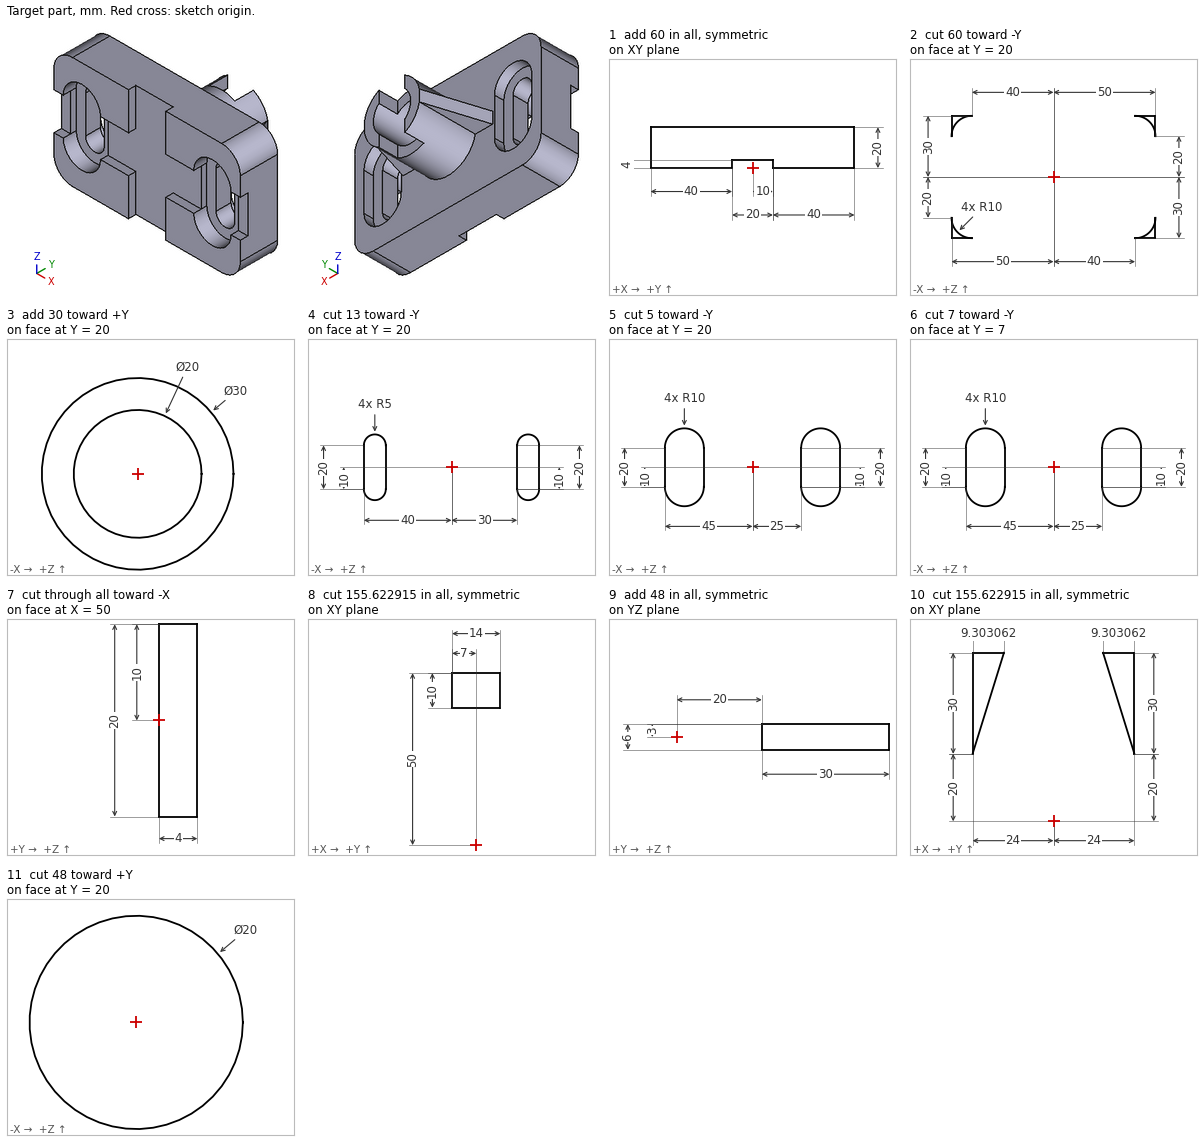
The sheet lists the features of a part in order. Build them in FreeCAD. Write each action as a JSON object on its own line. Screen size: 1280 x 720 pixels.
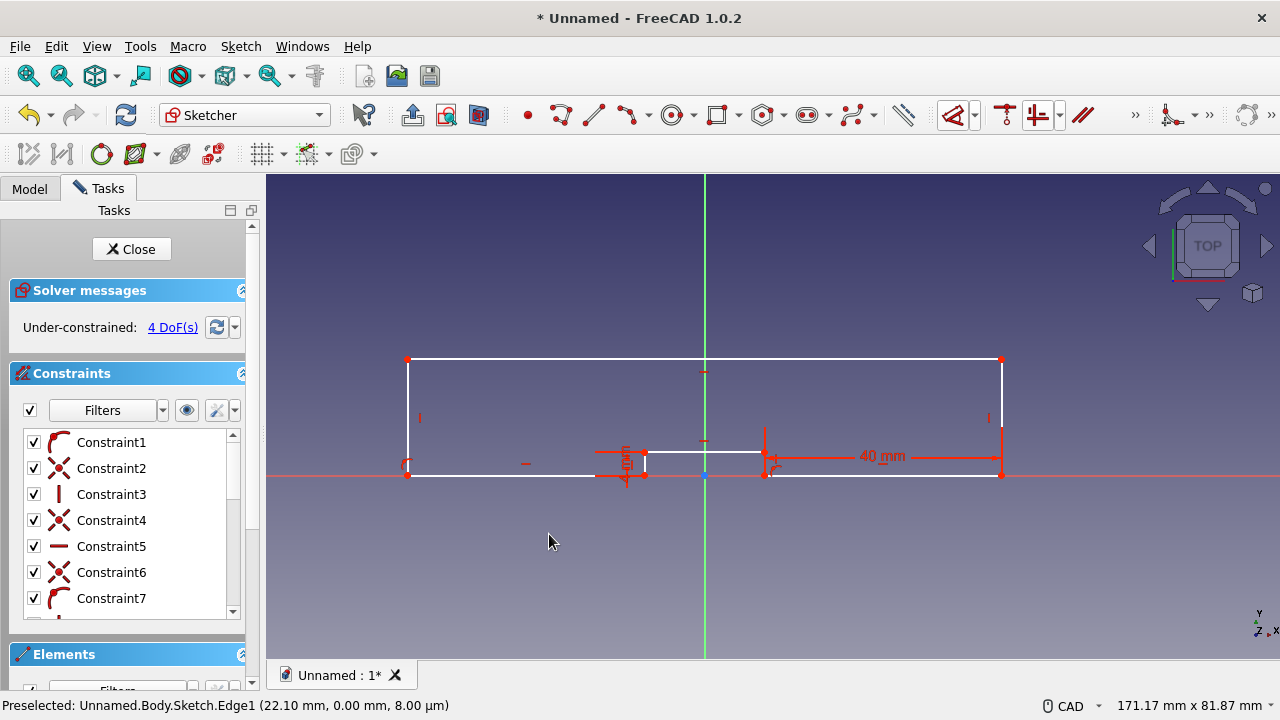
{"action": "left_click", "coordinate": [1002, 441]}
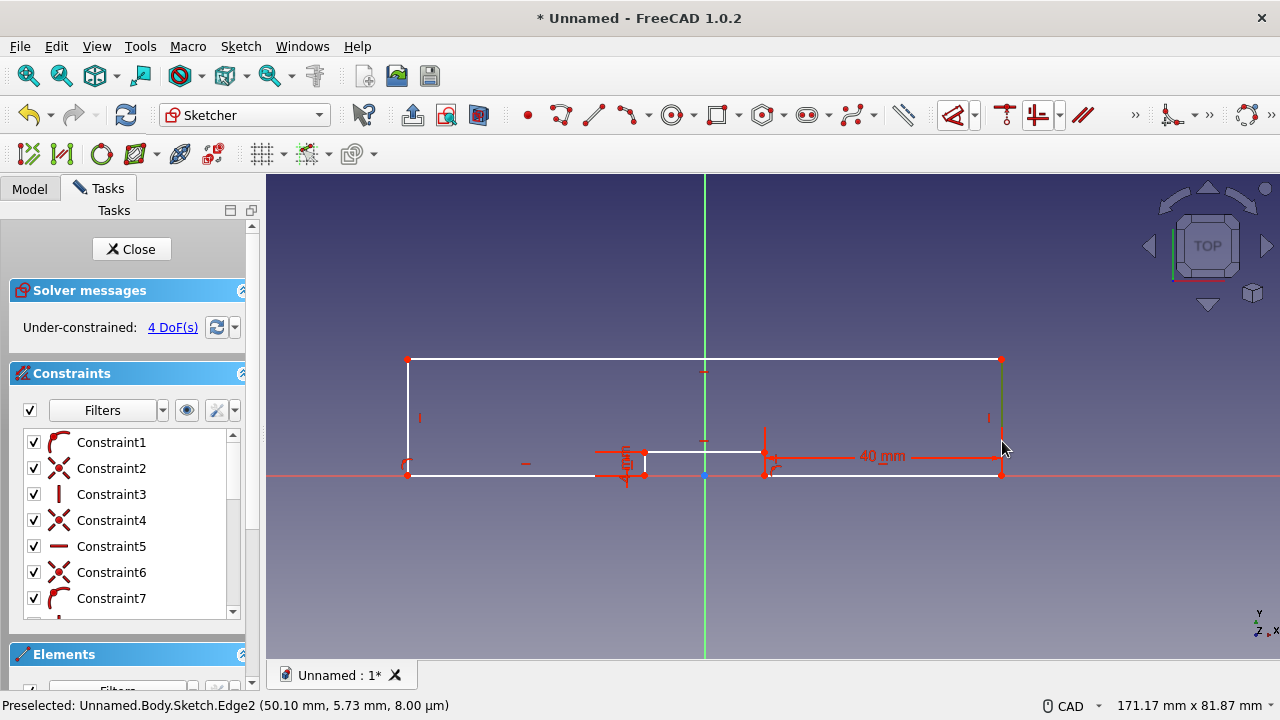
{"action": "key", "text": "i"}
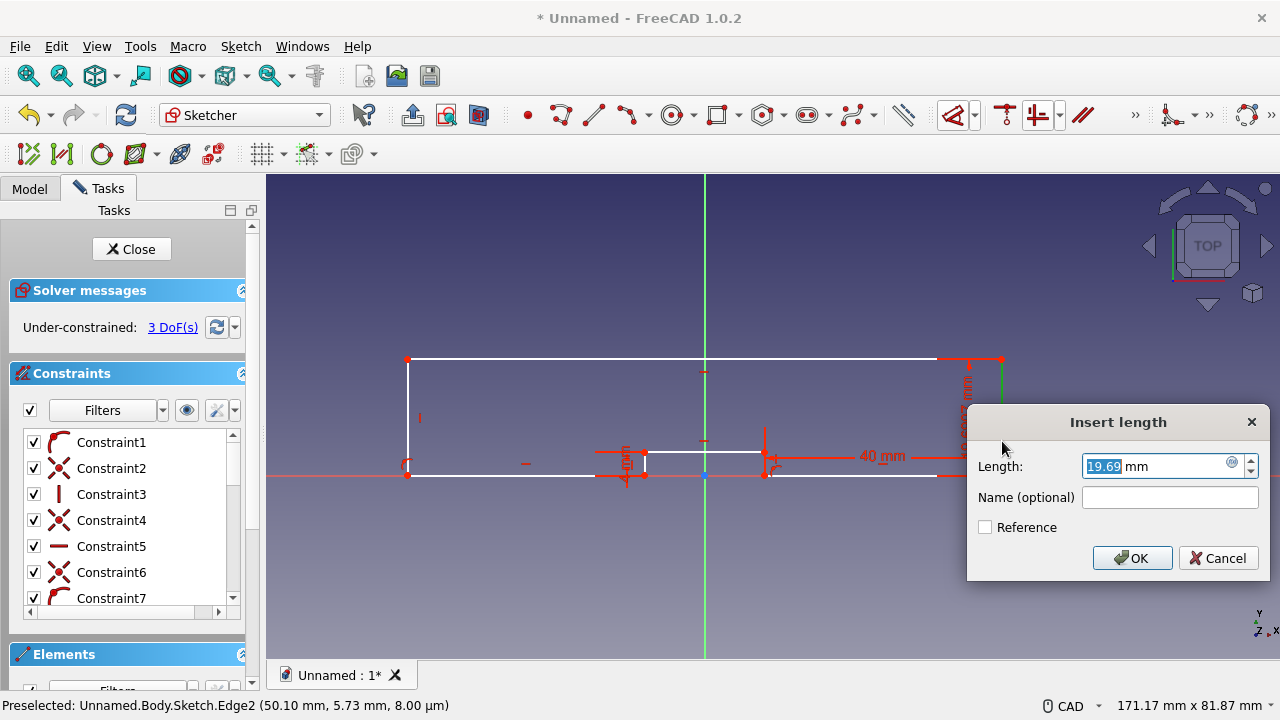
{"action": "type", "text": "20"}
{"action": "key", "text": "Return"}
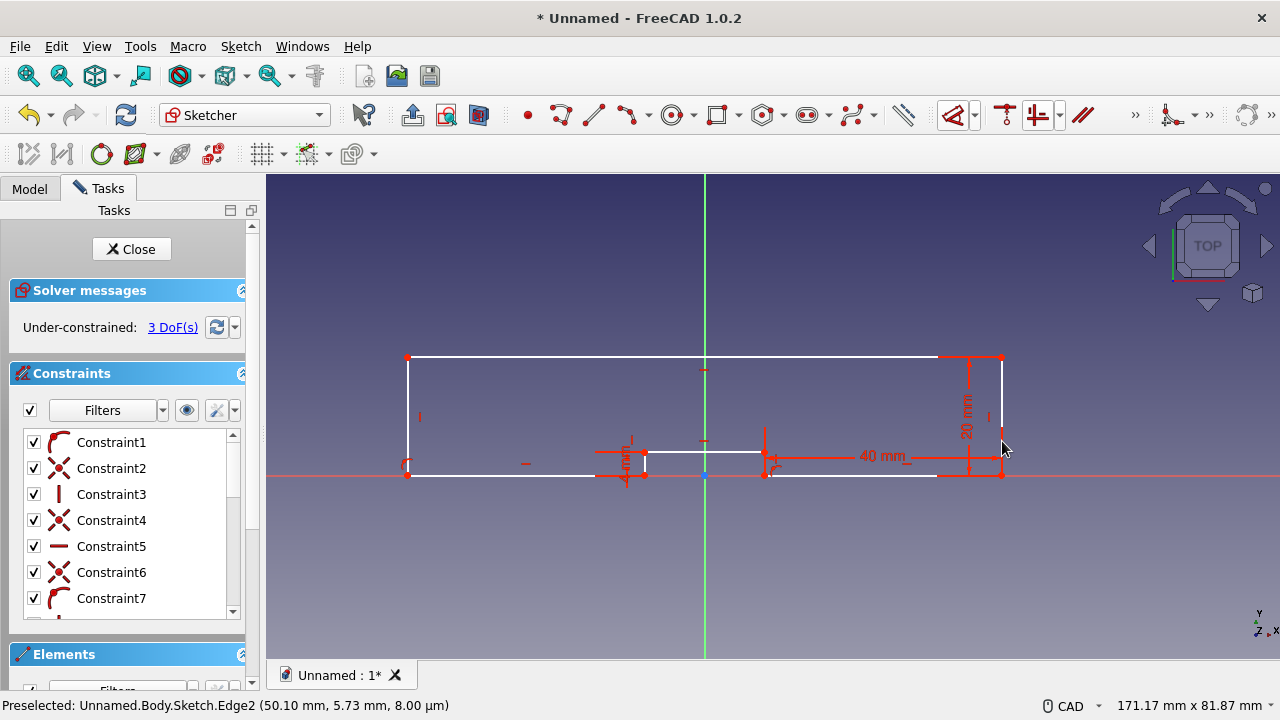
{"action": "left_click", "coordinate": [479, 476]}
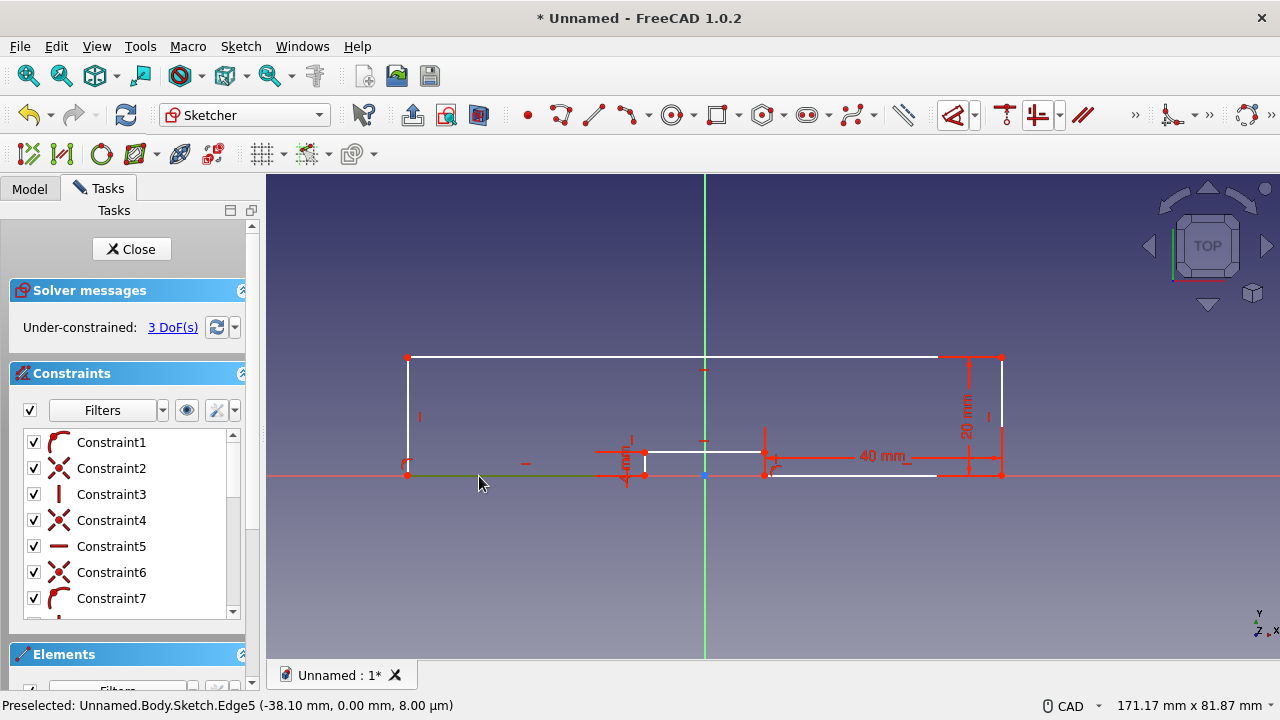
{"action": "left_click", "coordinate": [974, 116]}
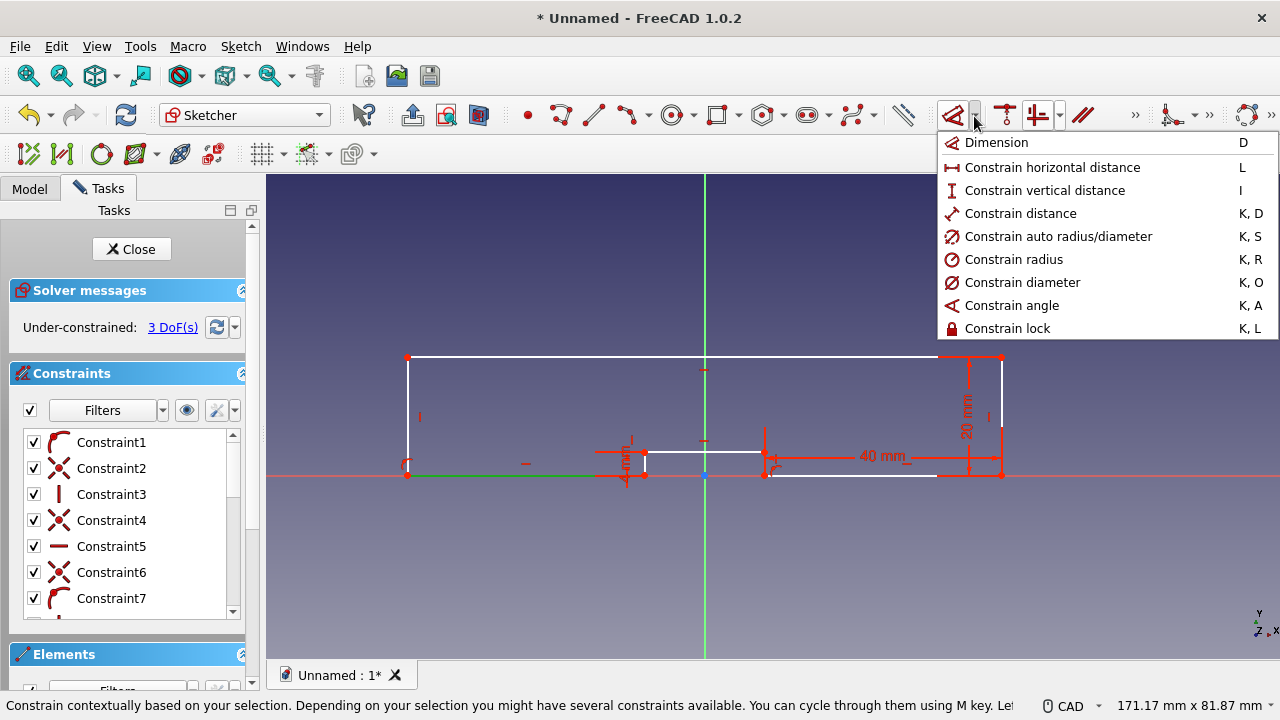
{"action": "left_click", "coordinate": [1108, 168]}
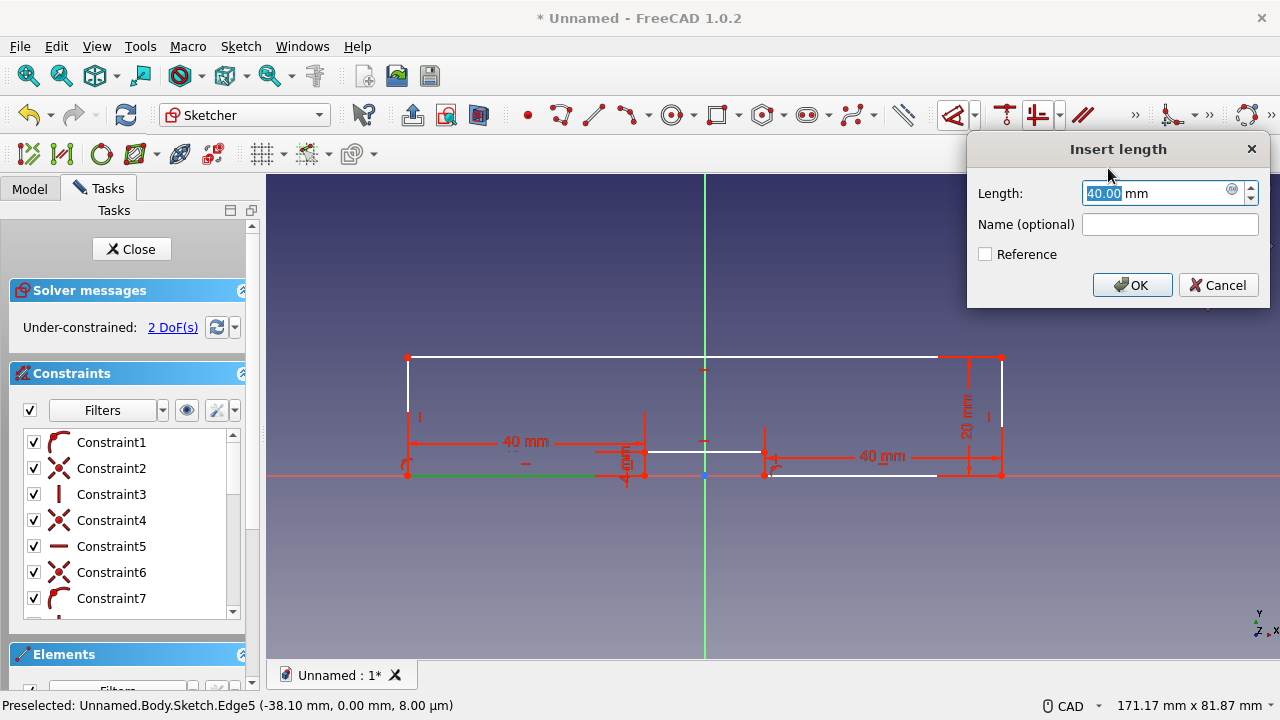
{"action": "type", "text": "40"}
{"action": "key", "text": "Return"}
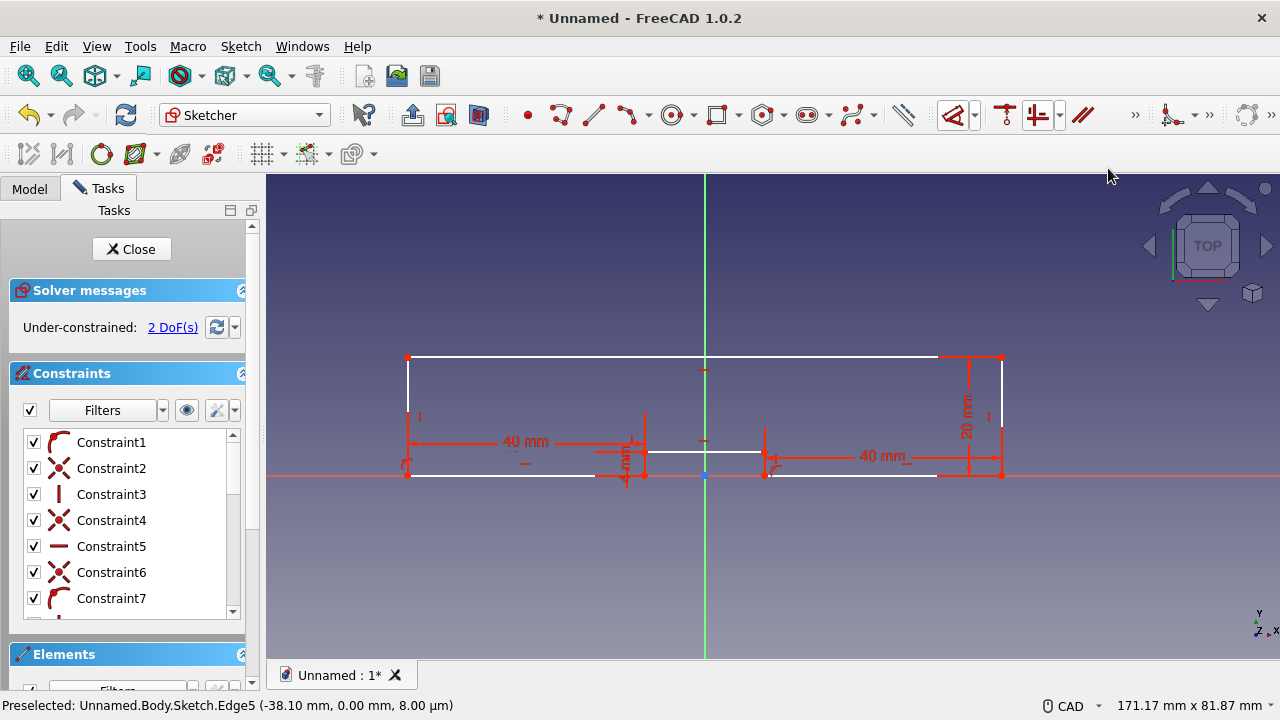
{"action": "left_click", "coordinate": [681, 452]}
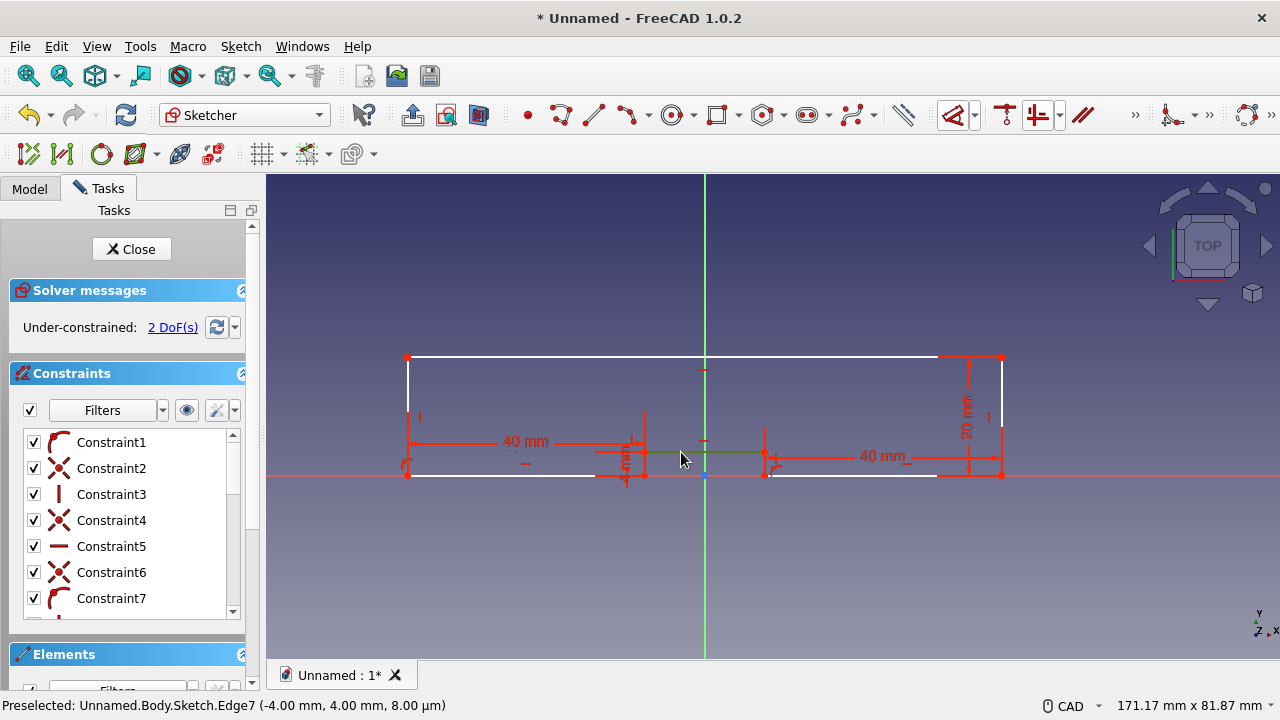
{"action": "key", "text": "l"}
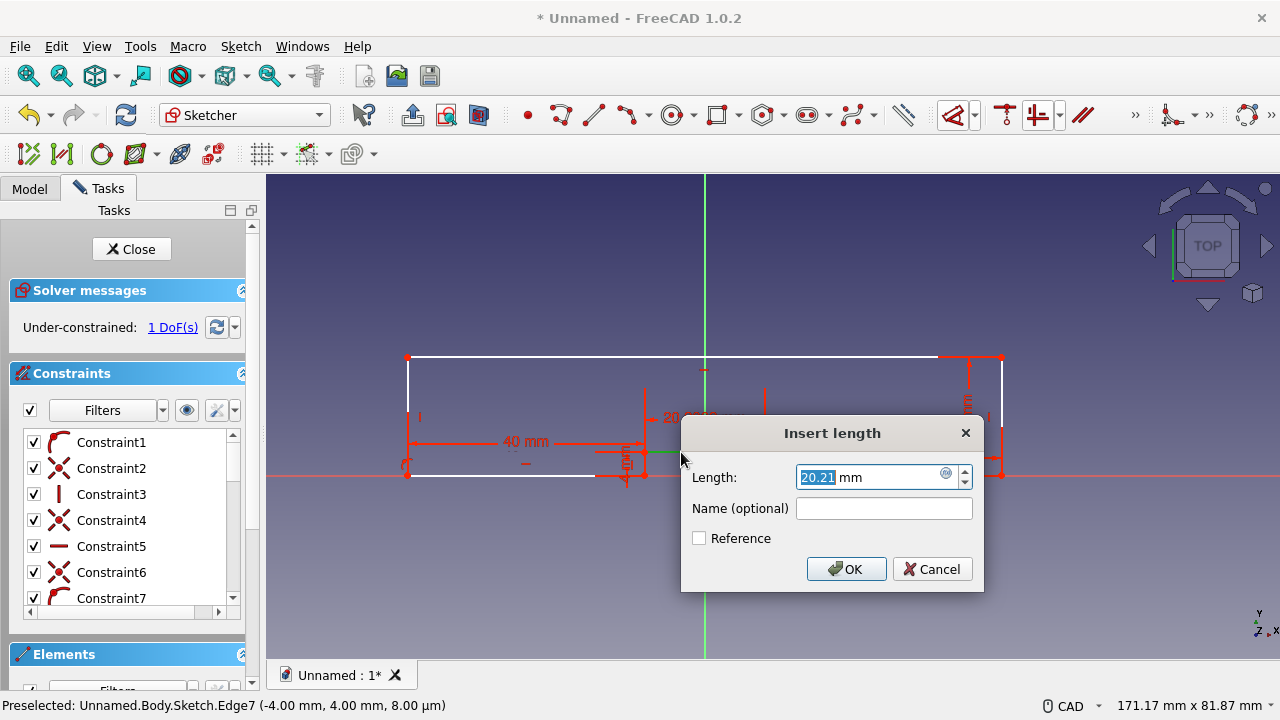
{"action": "type", "text": "20"}
{"action": "key", "text": "Return"}